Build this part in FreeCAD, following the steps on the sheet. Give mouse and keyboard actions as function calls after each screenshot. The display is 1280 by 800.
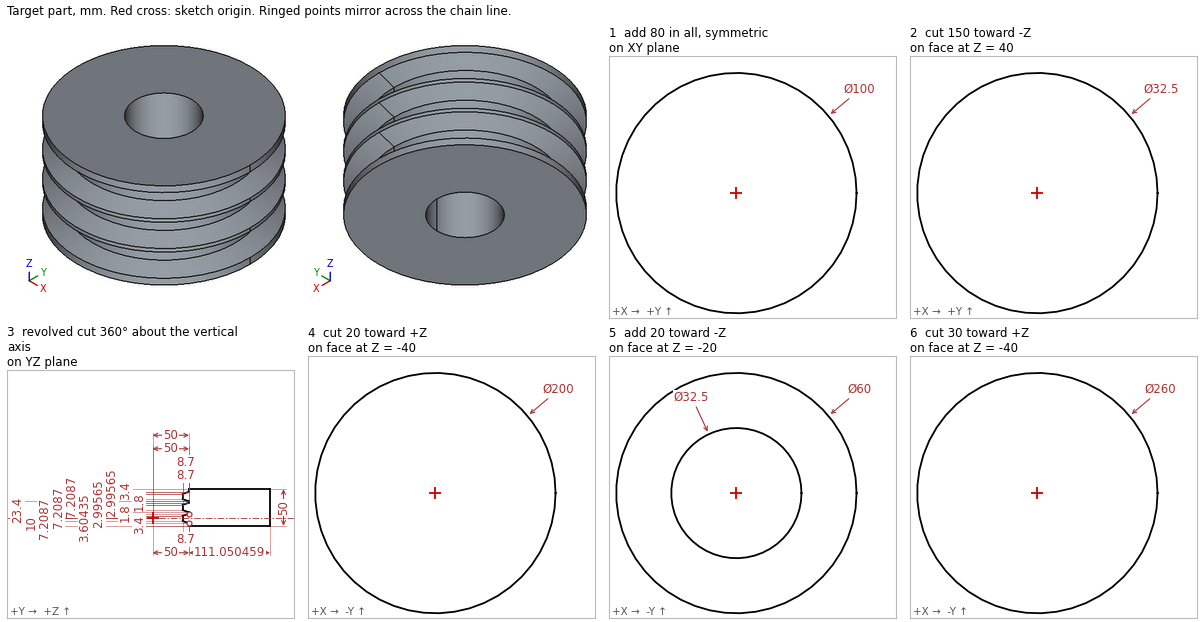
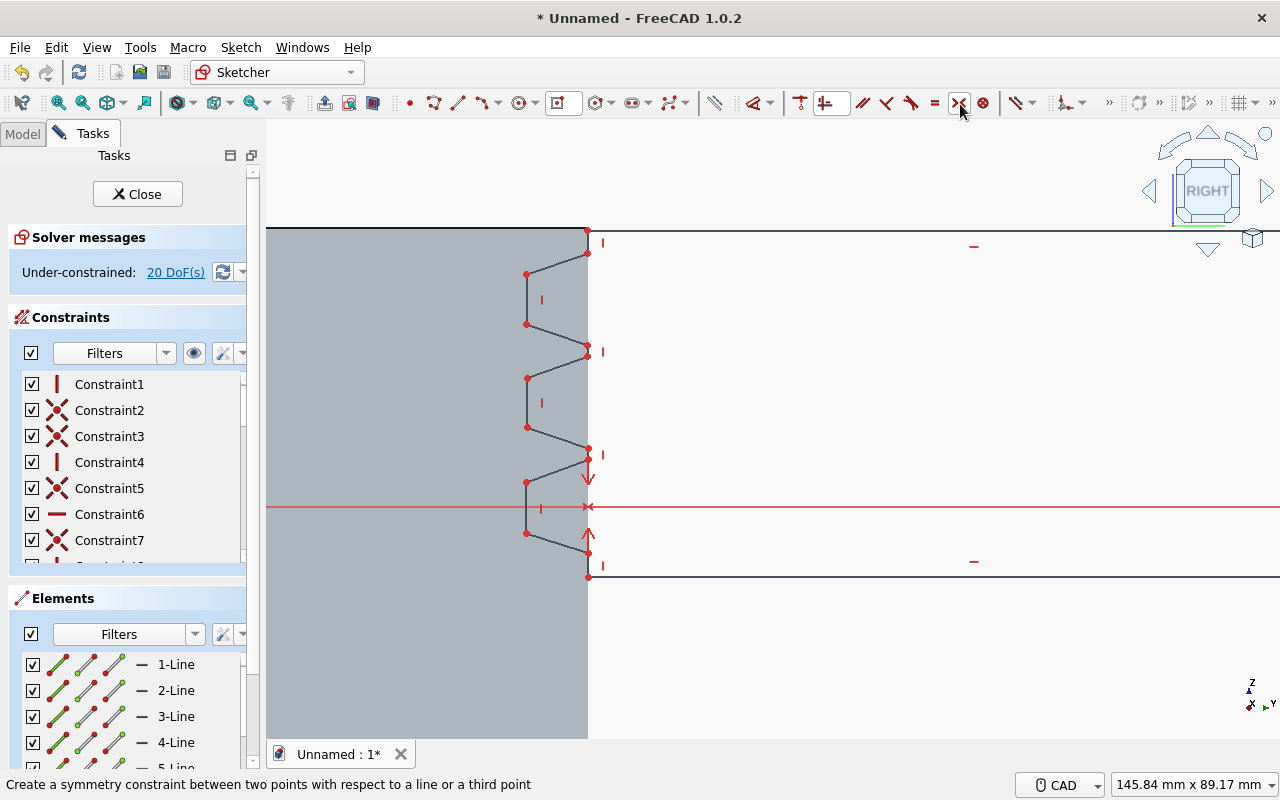
click(754, 104)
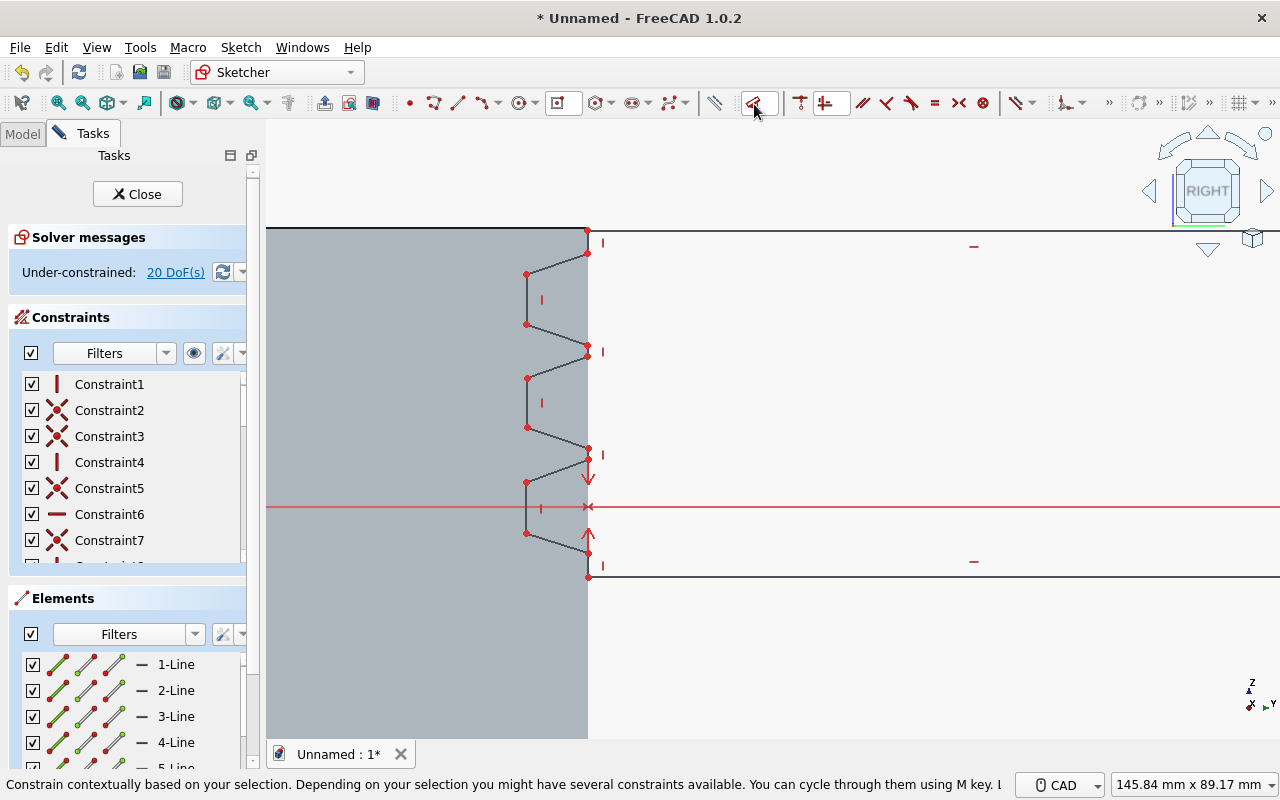
scroll(588, 462, down, 3)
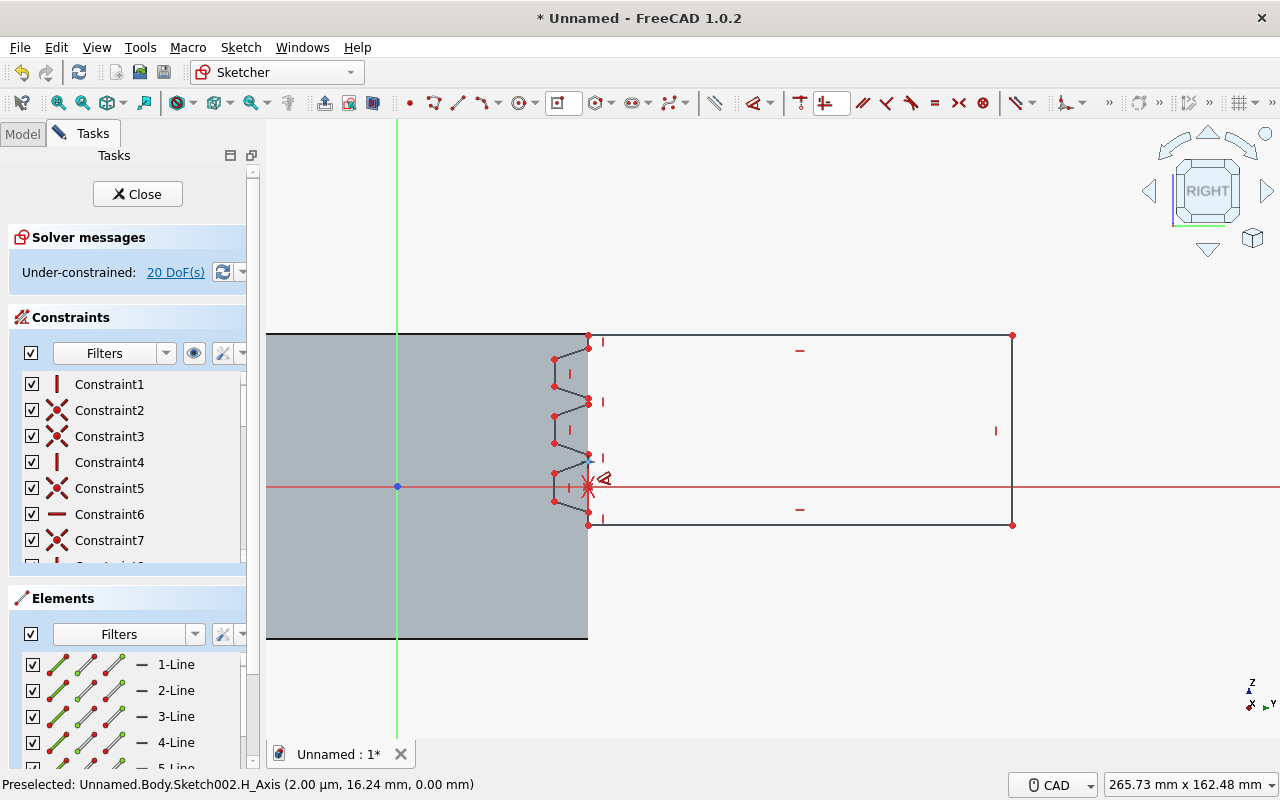
click(1012, 468)
click(1046, 430)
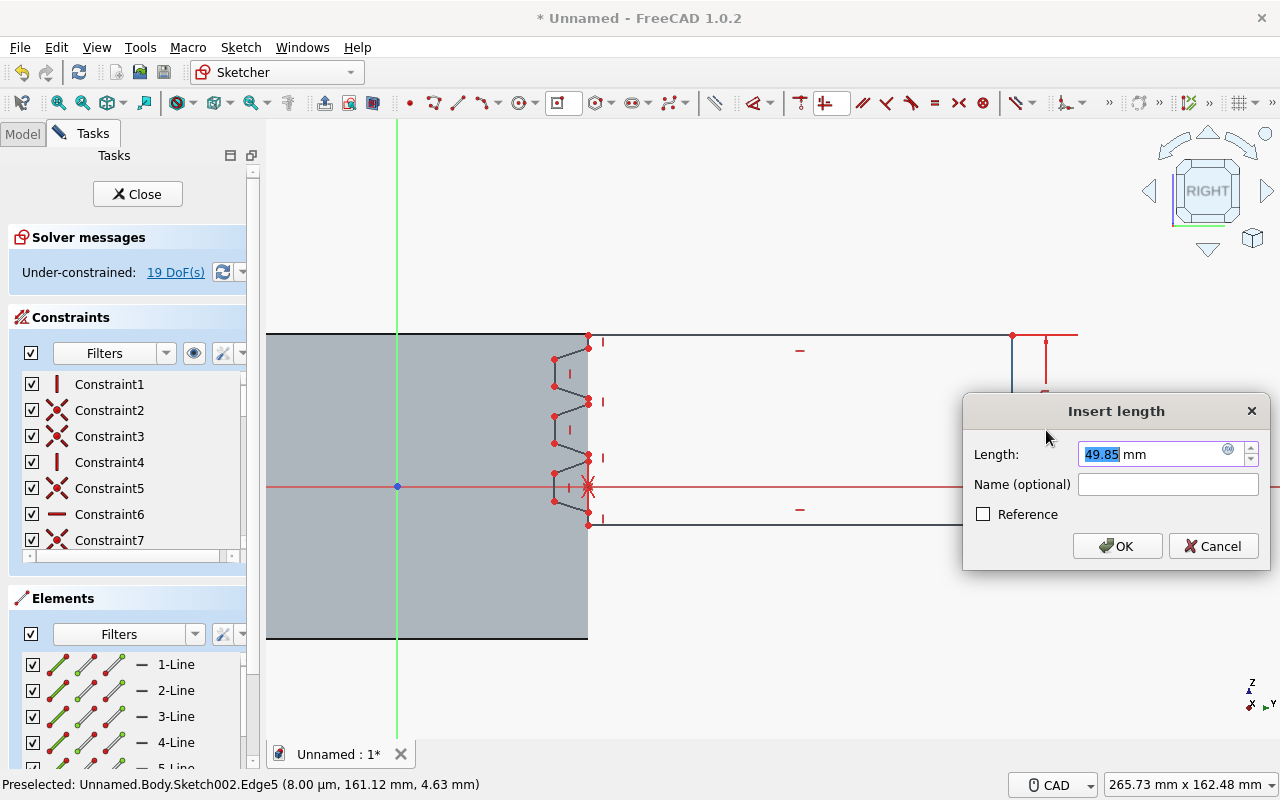
text(50)
key(Return)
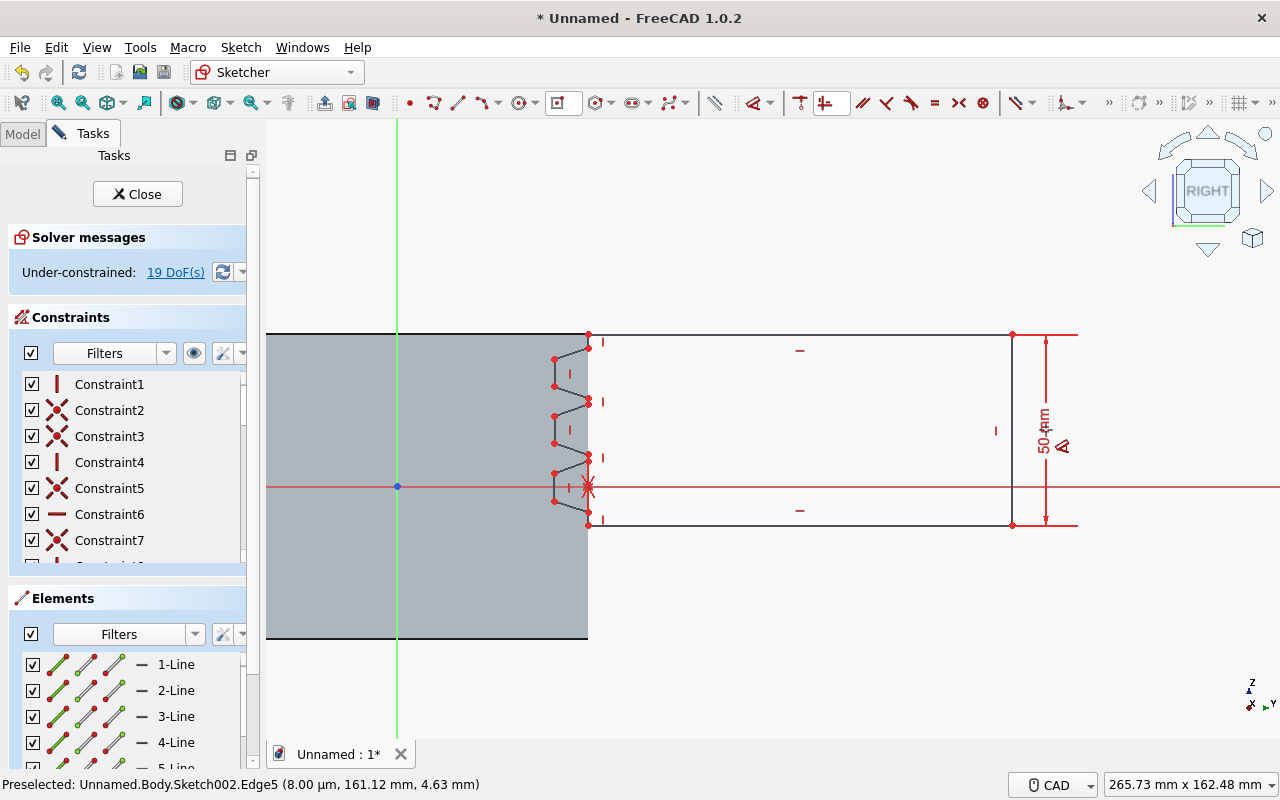
scroll(588, 519, up, 6)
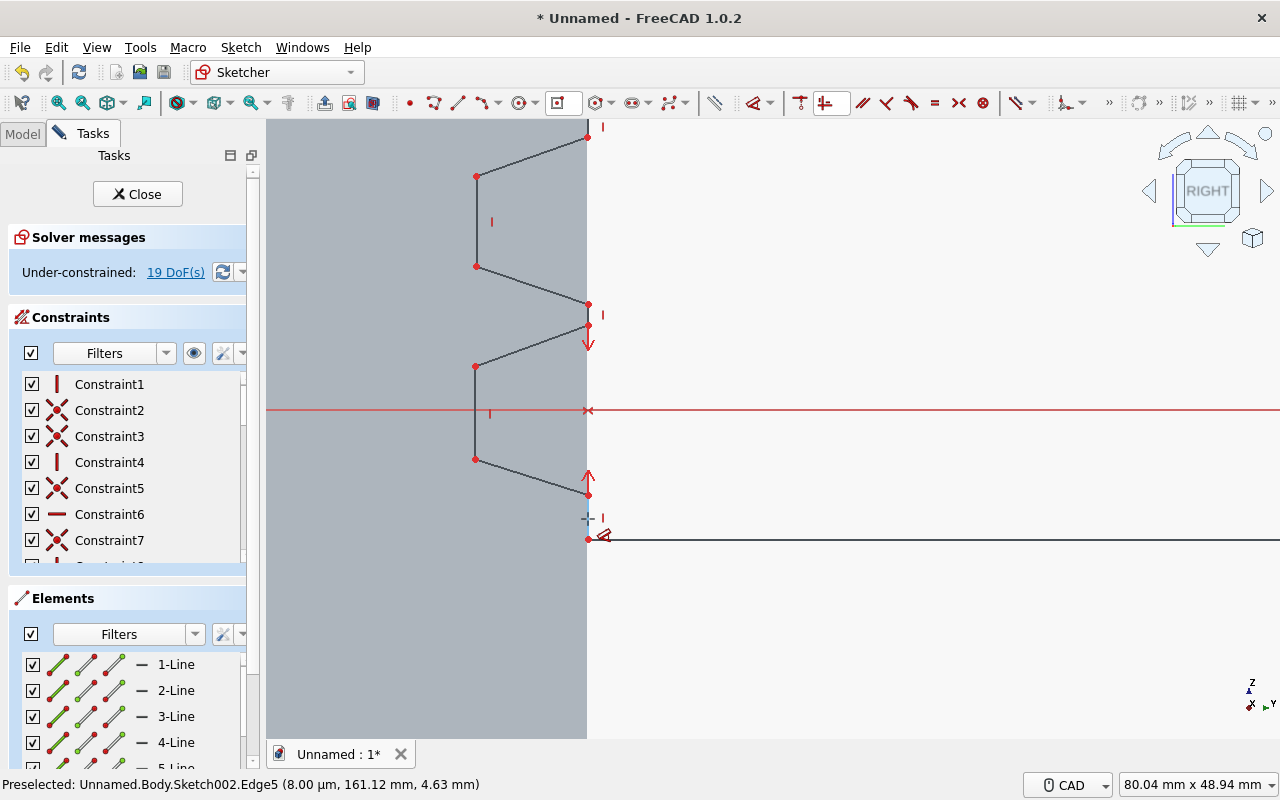
click(588, 518)
click(554, 518)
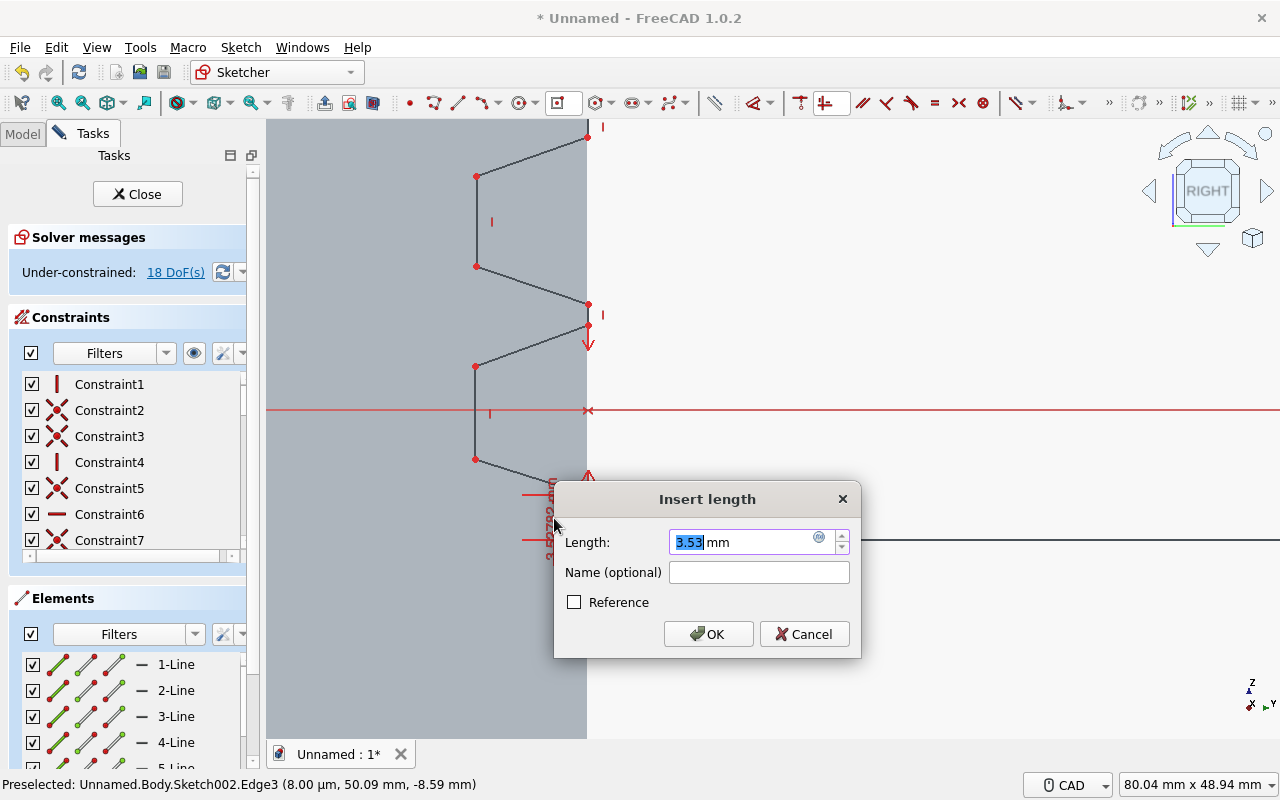
text(3.4)
key(Return)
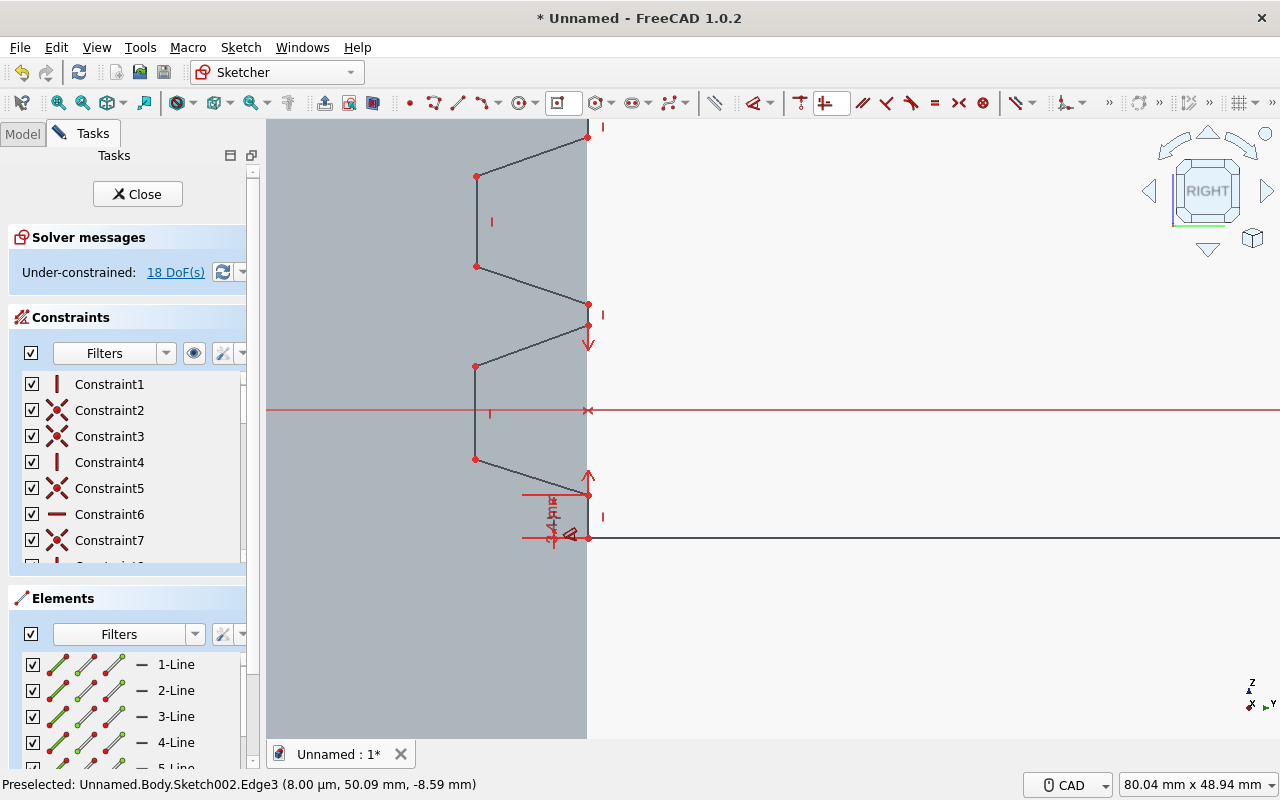
scroll(588, 519, down, 6)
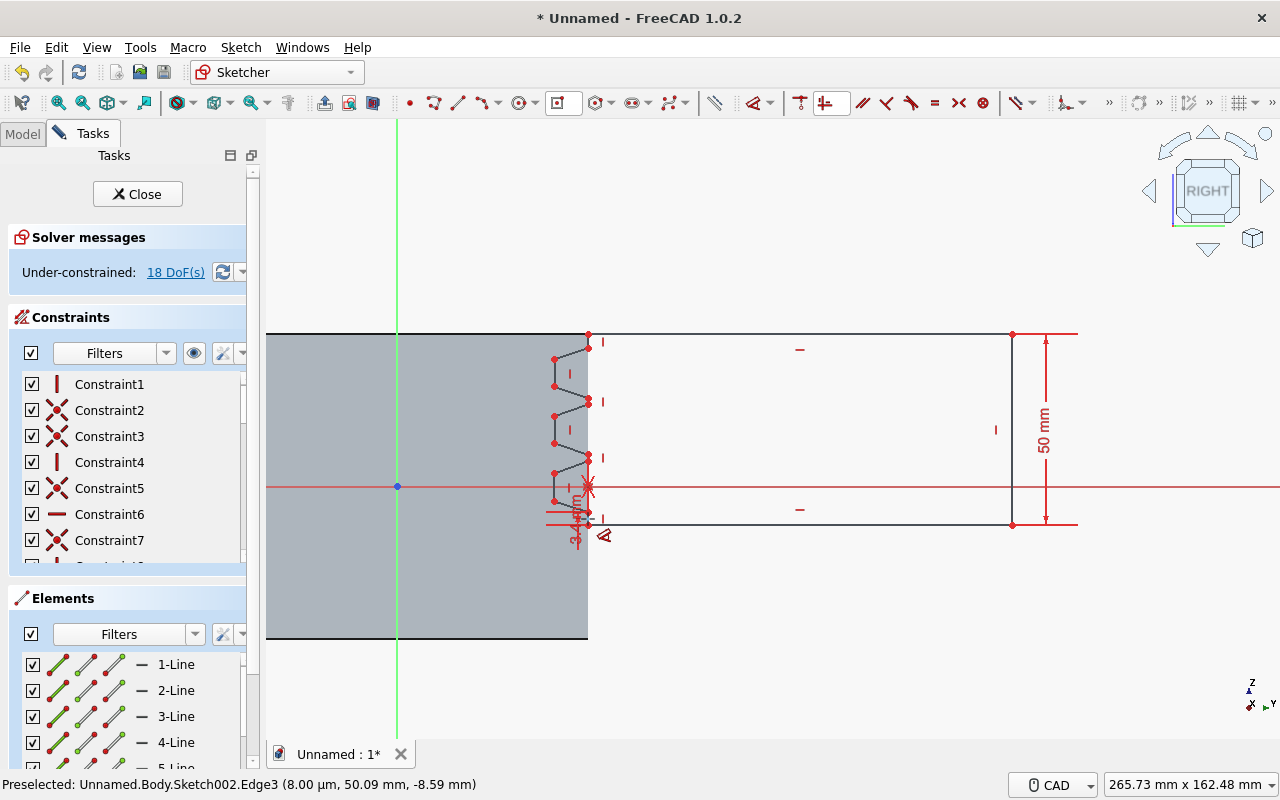
scroll(588, 339, up, 7)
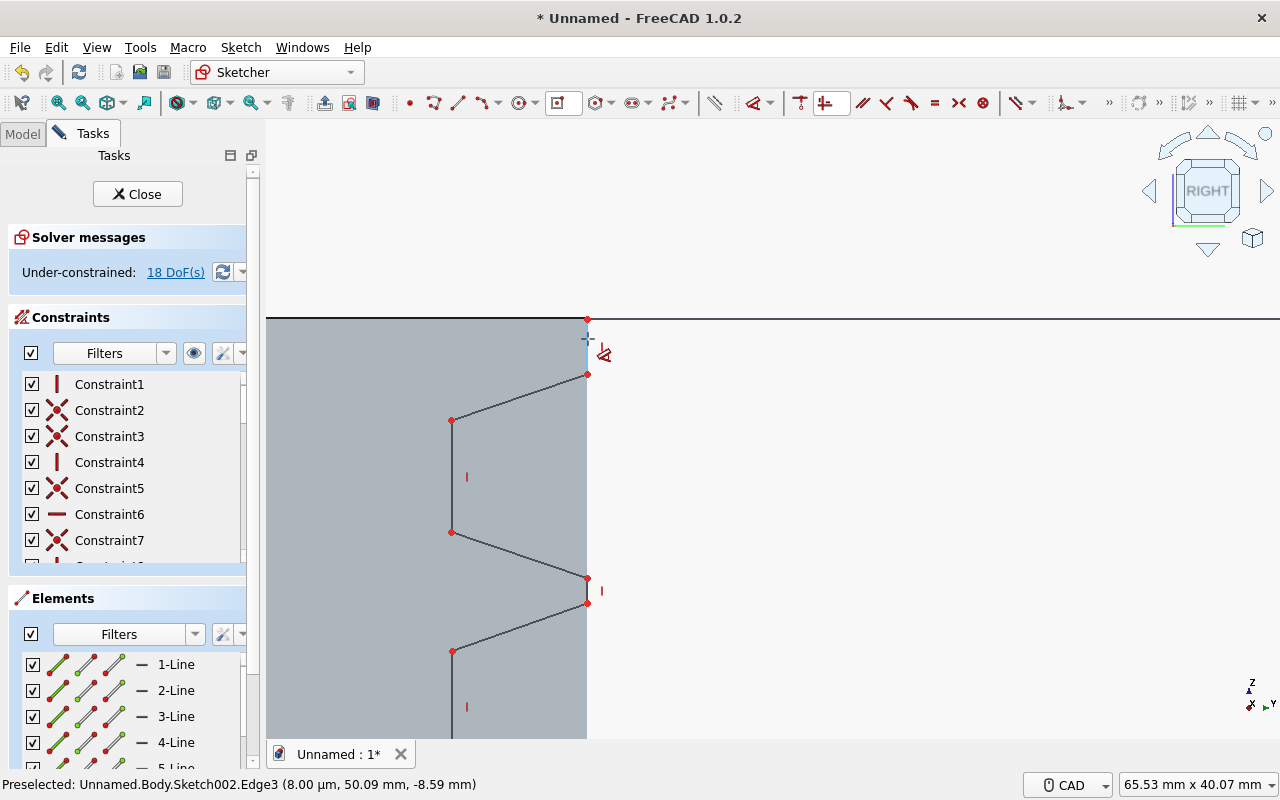
click(587, 336)
click(553, 347)